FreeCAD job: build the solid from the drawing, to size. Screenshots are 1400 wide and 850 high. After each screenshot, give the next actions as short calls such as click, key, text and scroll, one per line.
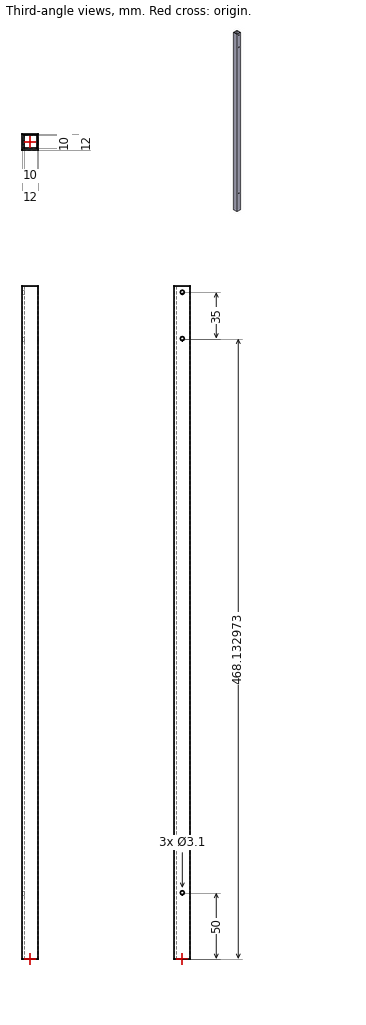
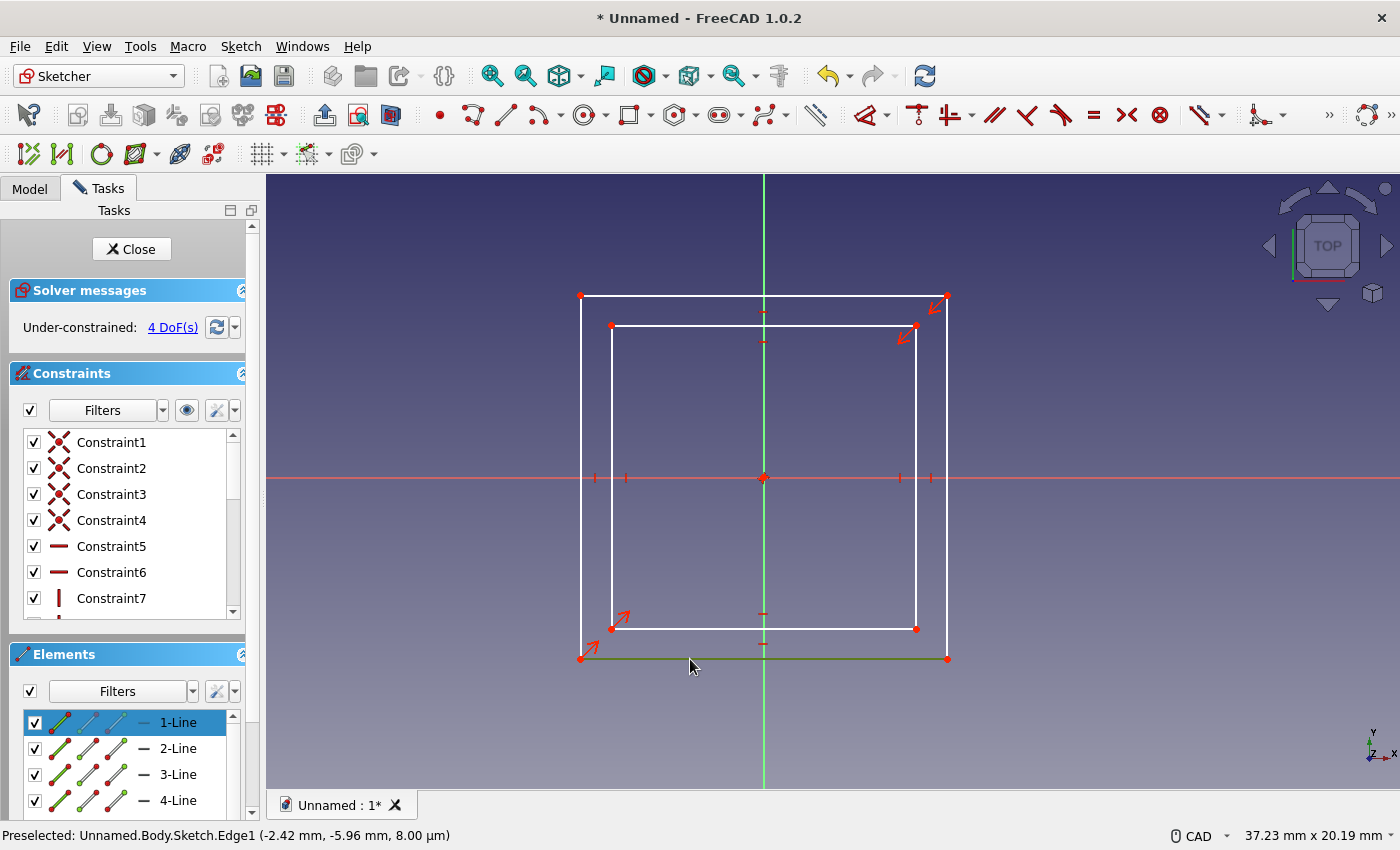
click(886, 116)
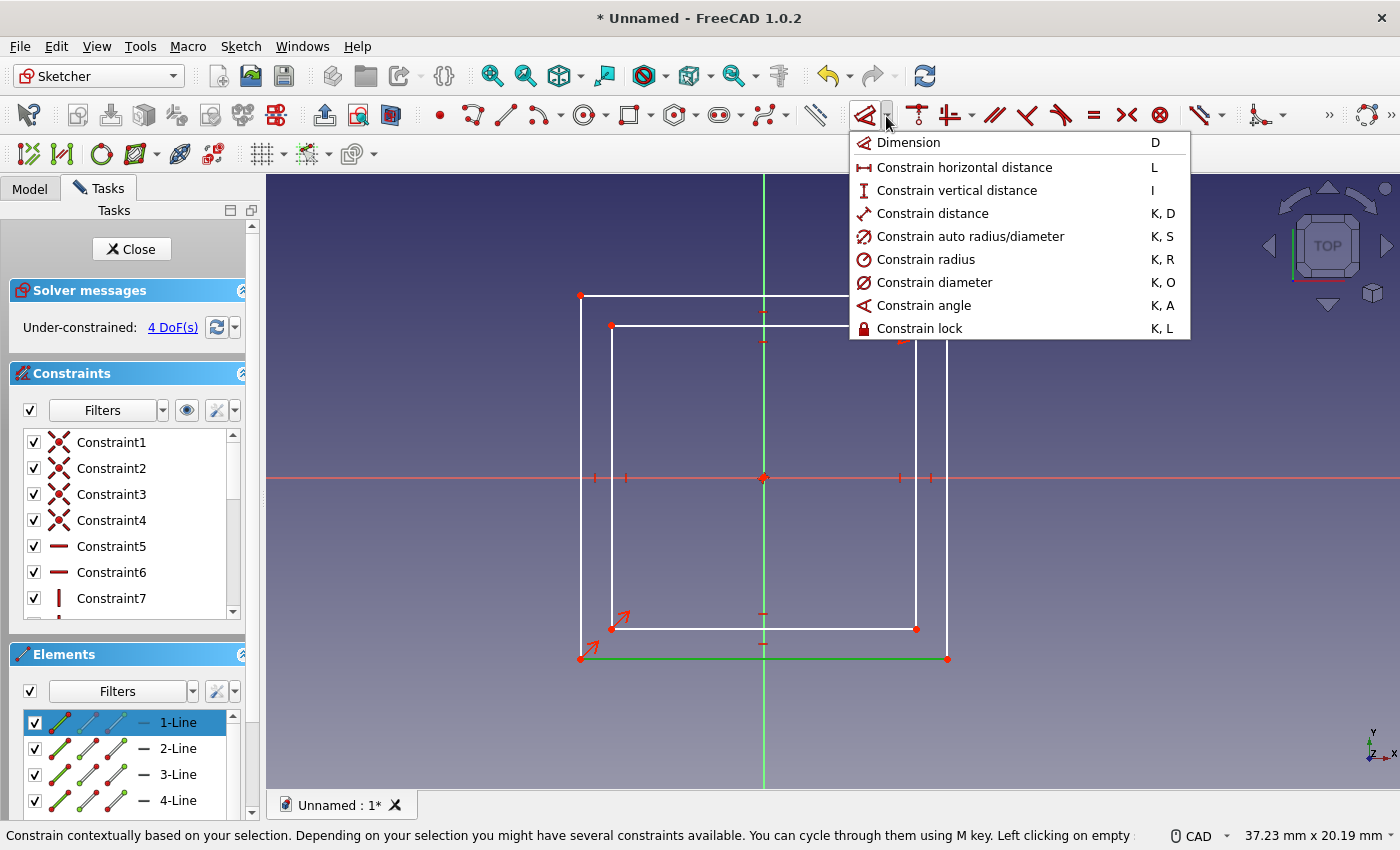
click(1020, 168)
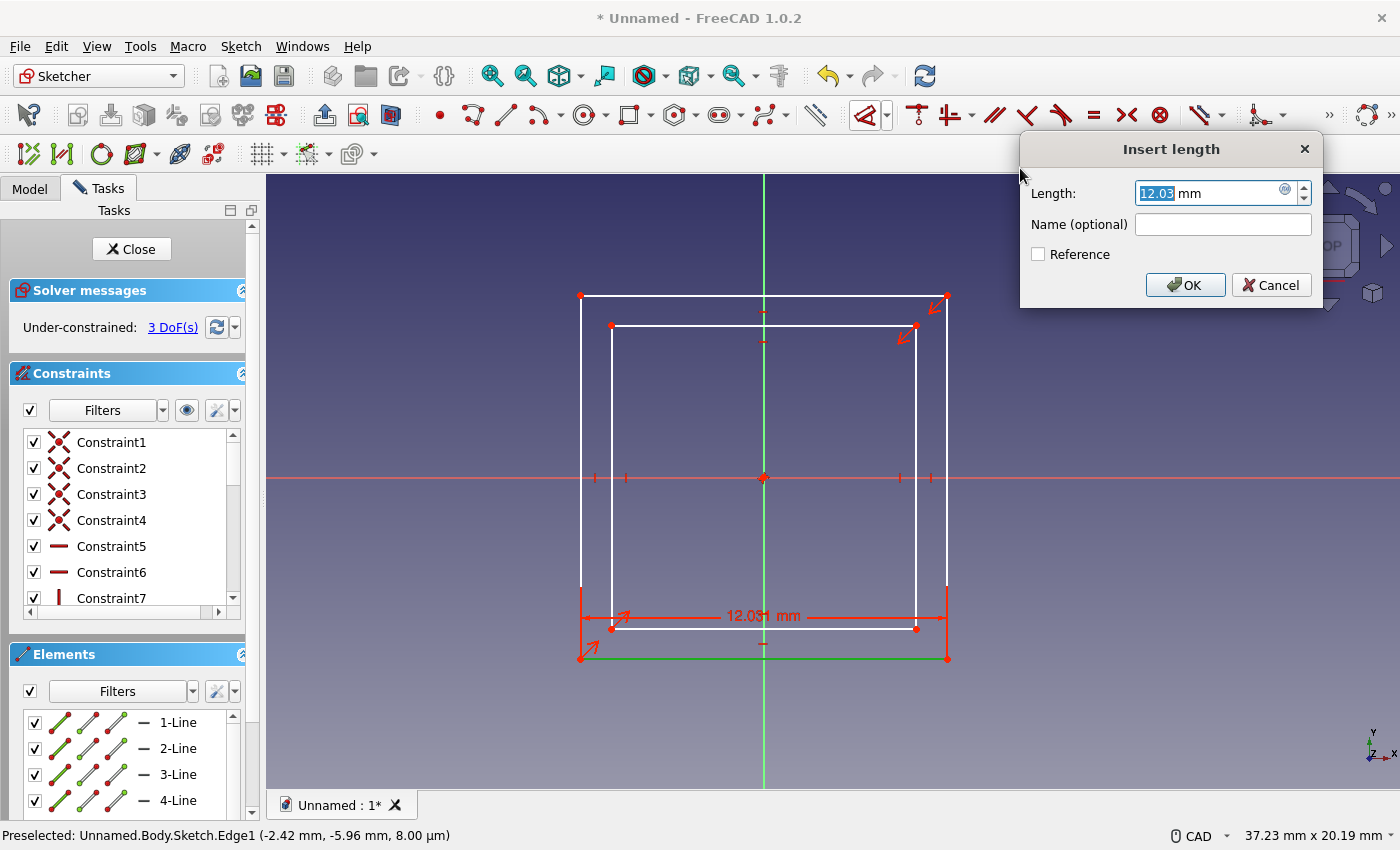
text(12)
key(Return)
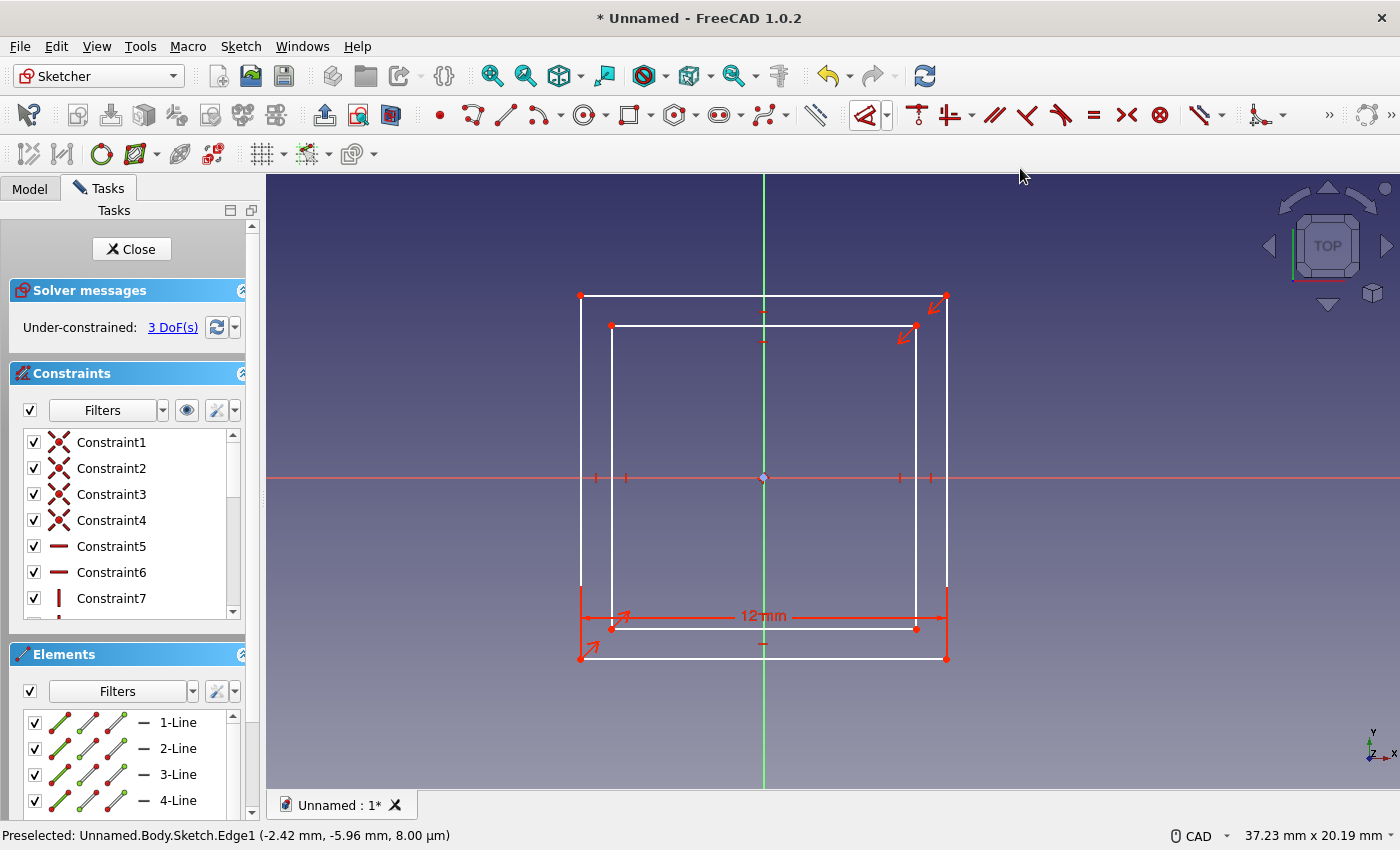
click(947, 550)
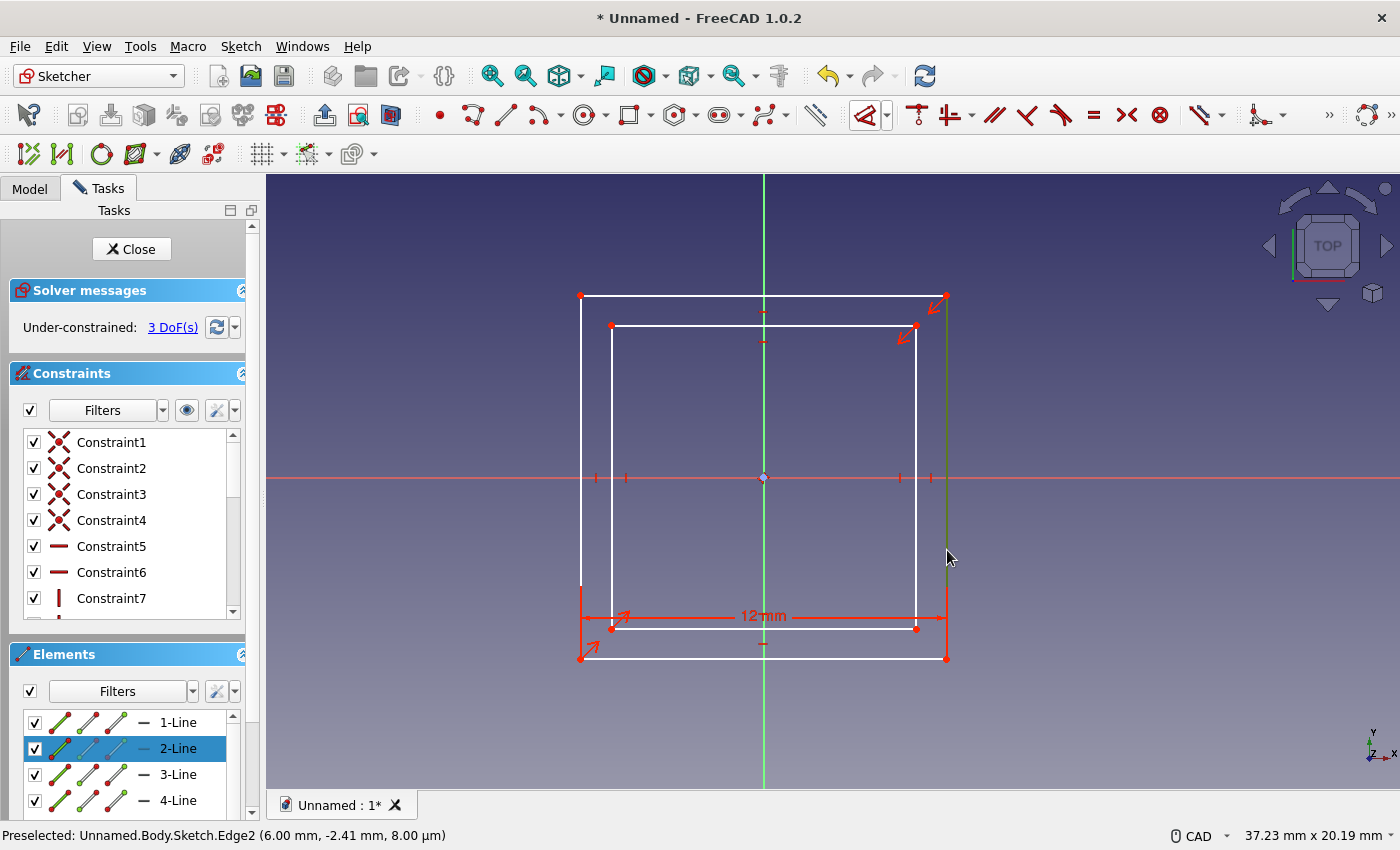
key(i)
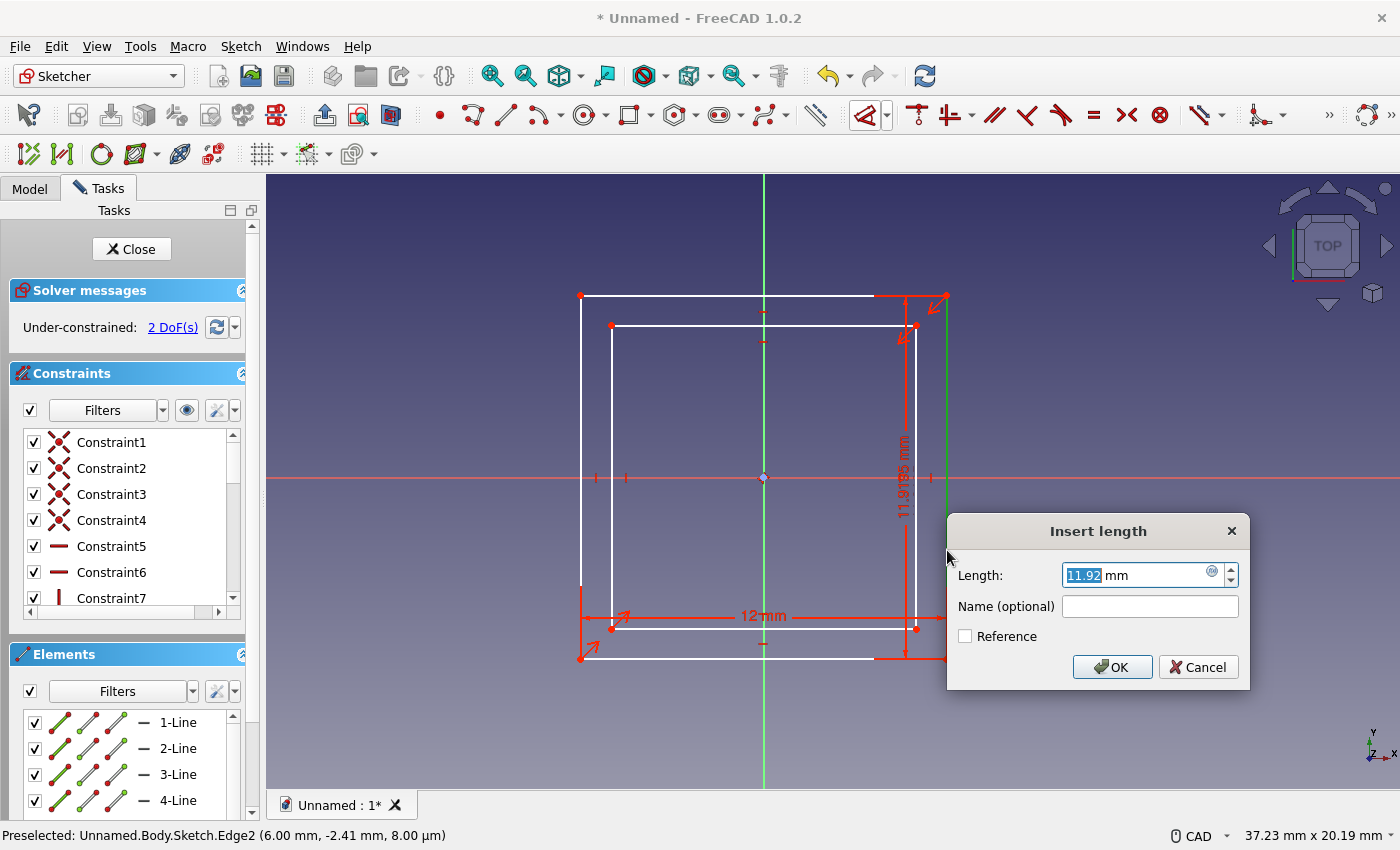
text(12)
key(Return)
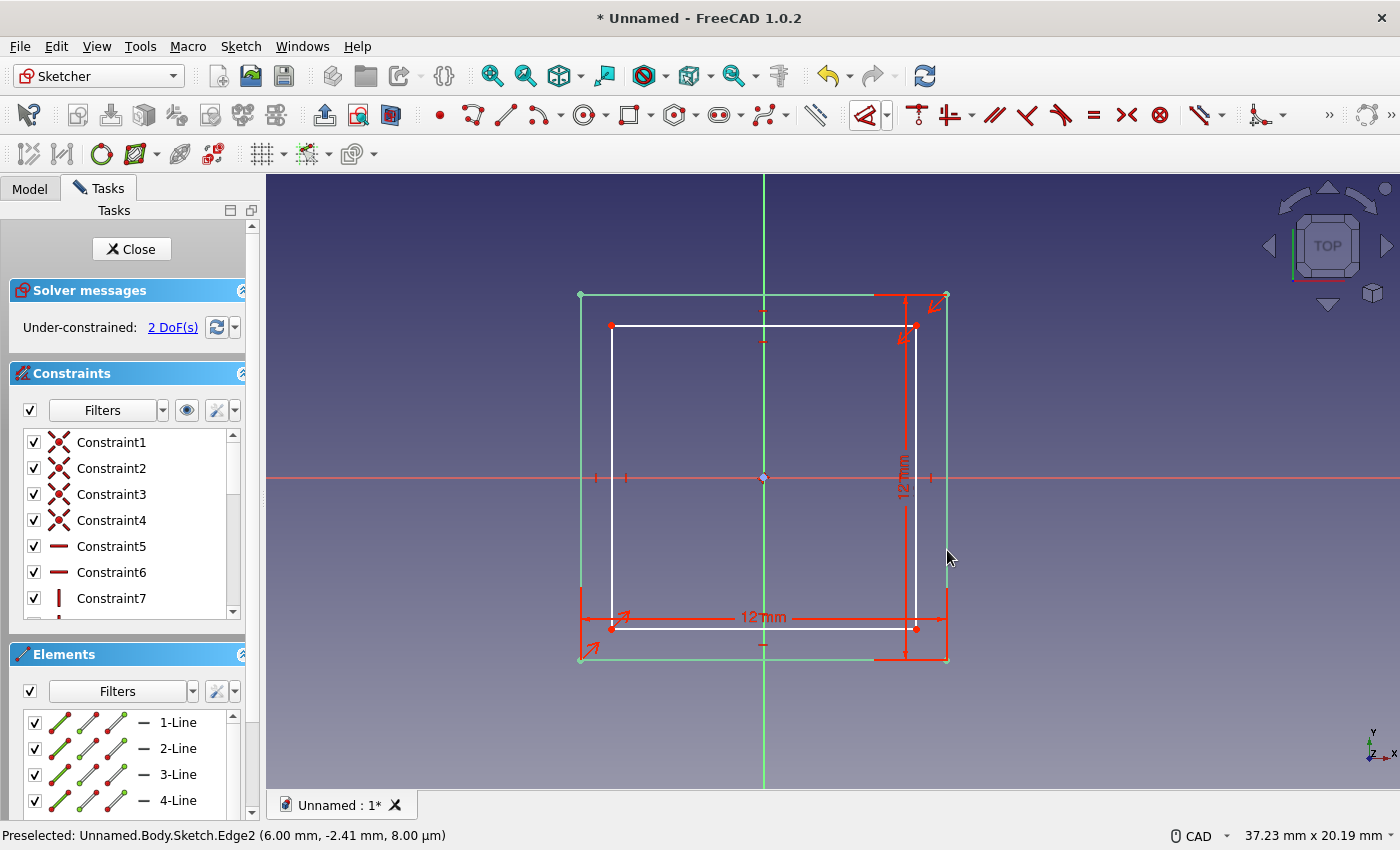
click(703, 629)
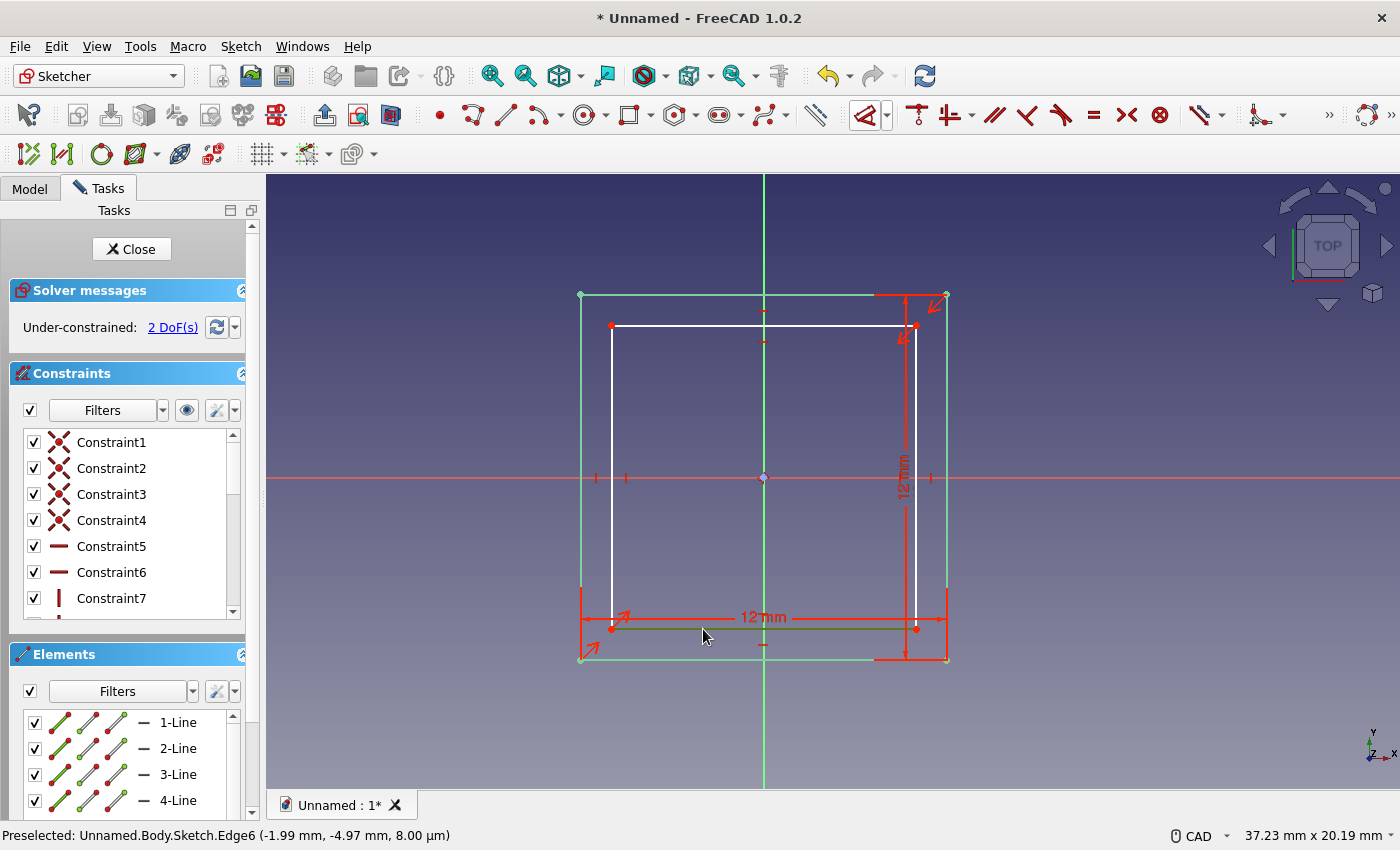
click(886, 116)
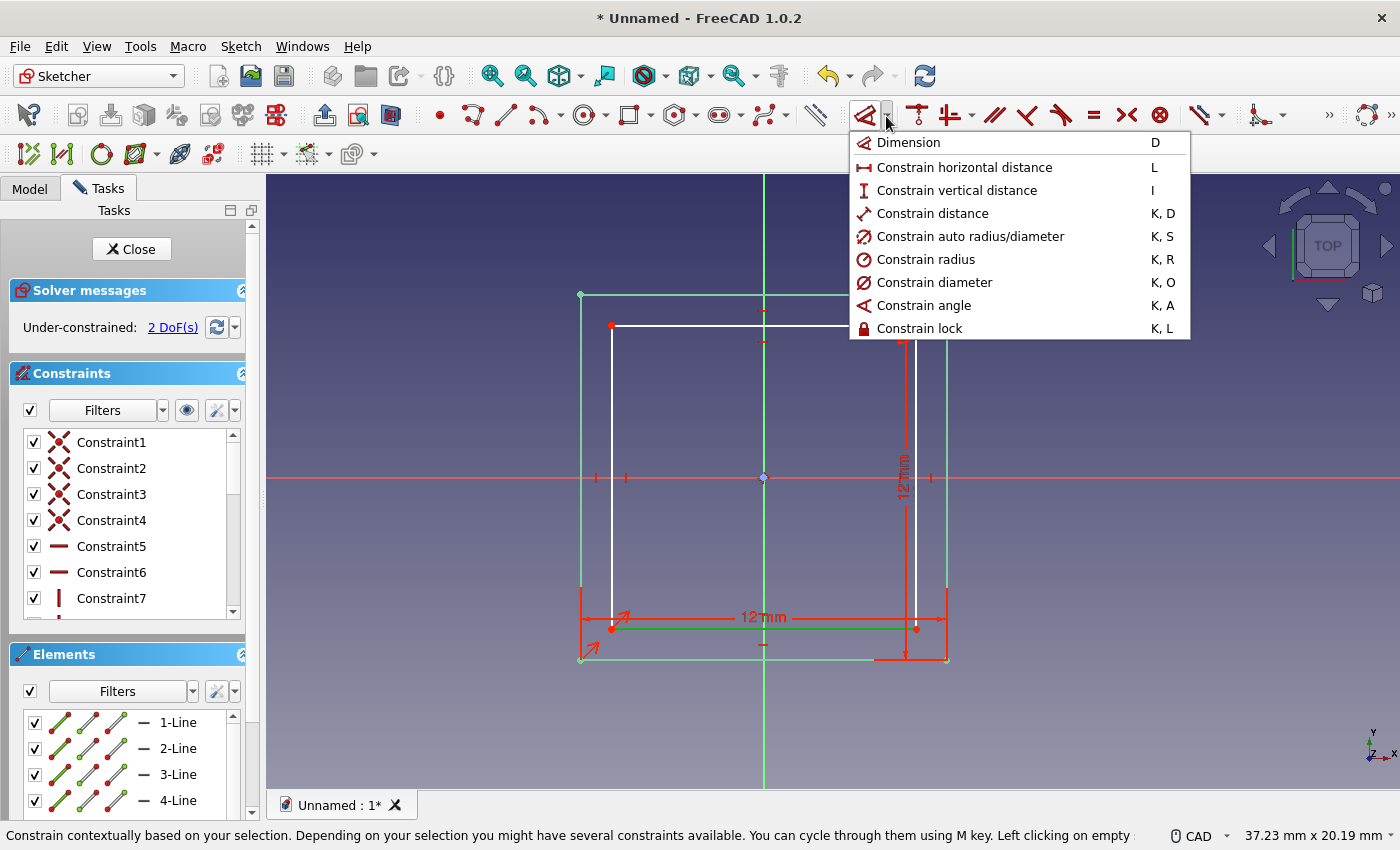
click(1020, 168)